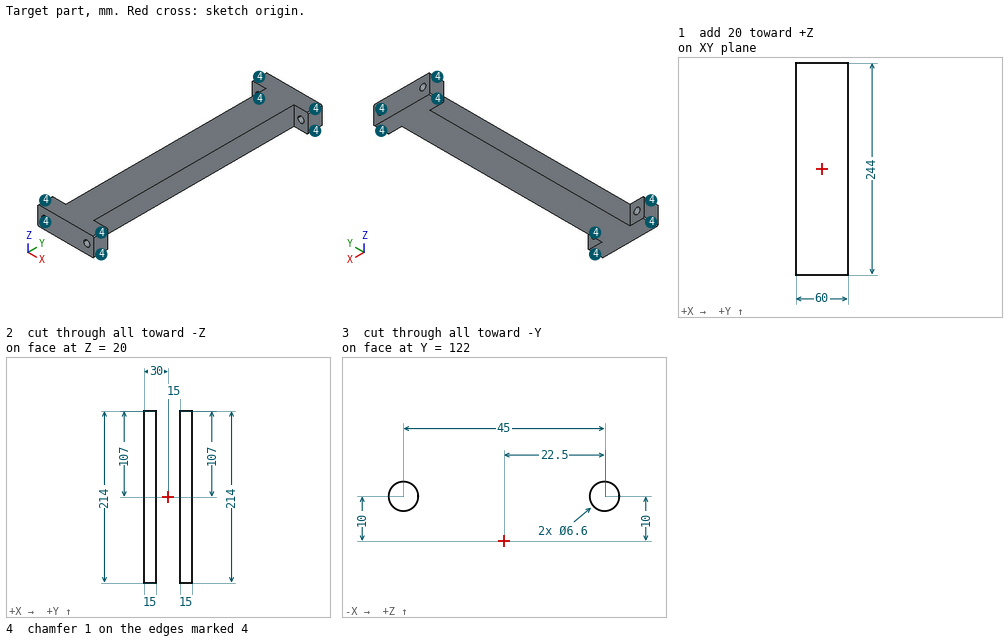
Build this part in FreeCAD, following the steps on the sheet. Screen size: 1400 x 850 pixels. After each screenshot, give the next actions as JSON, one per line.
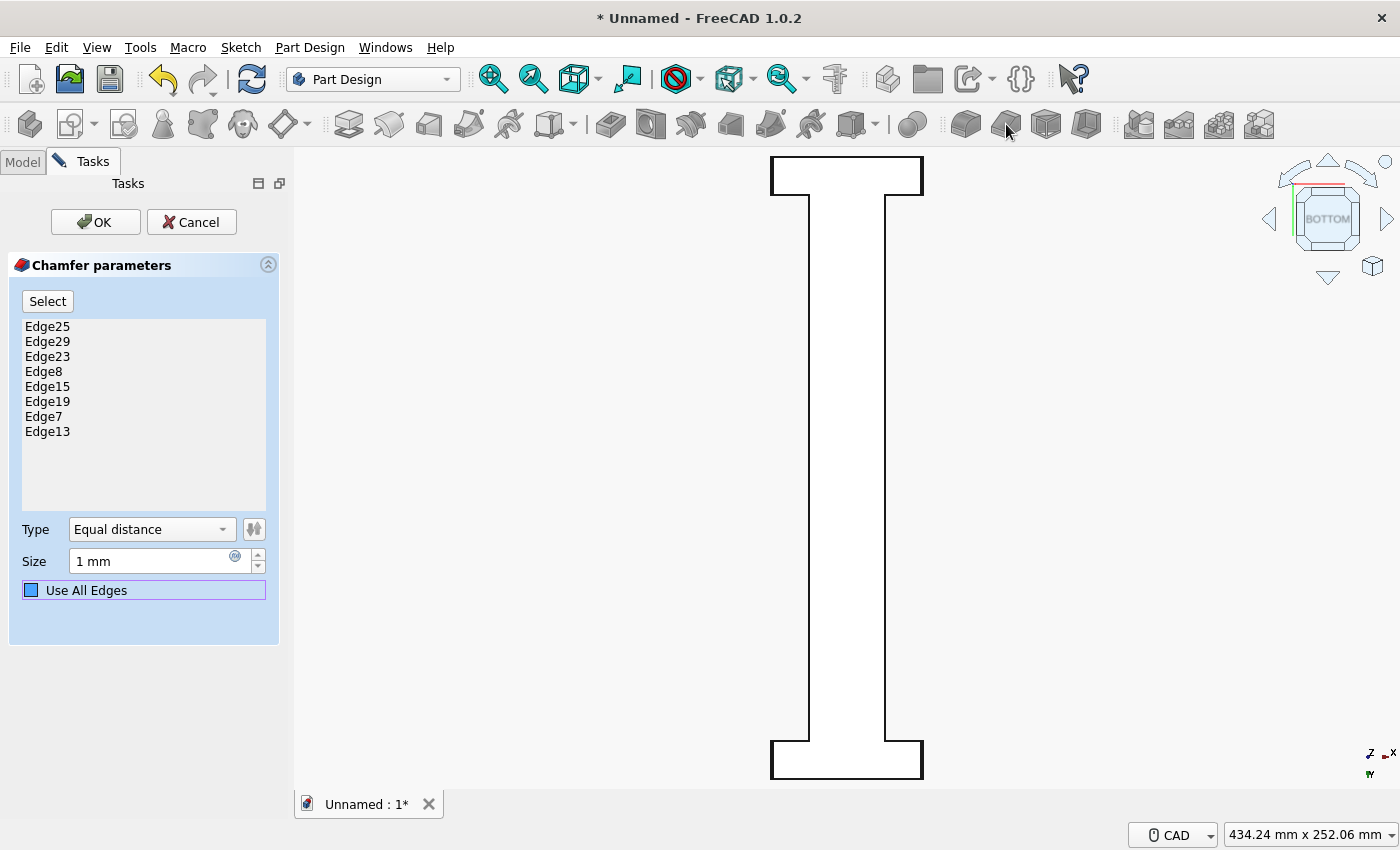
{"action": "left_click", "coordinate": [96, 222]}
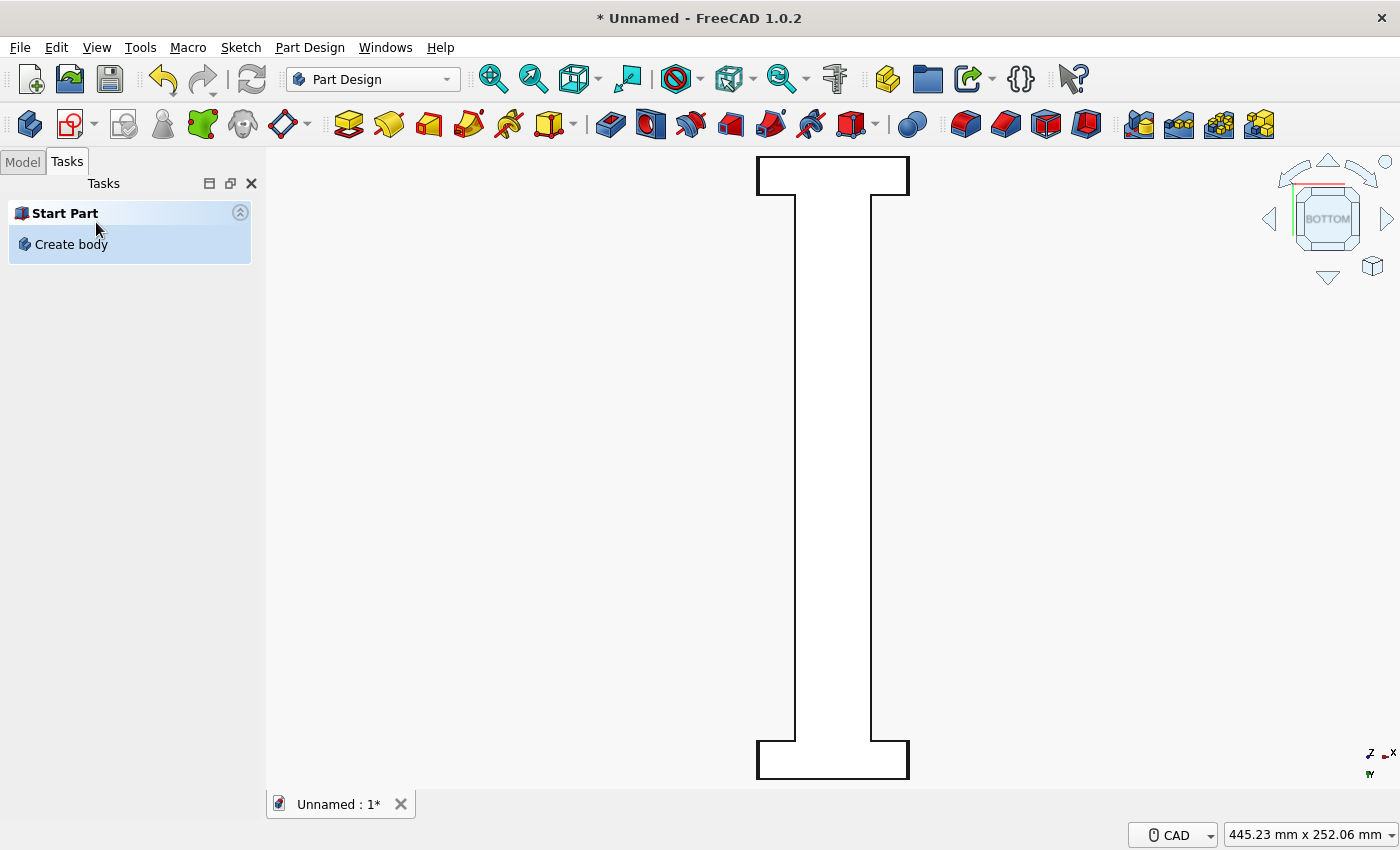
{"action": "key", "text": "0"}